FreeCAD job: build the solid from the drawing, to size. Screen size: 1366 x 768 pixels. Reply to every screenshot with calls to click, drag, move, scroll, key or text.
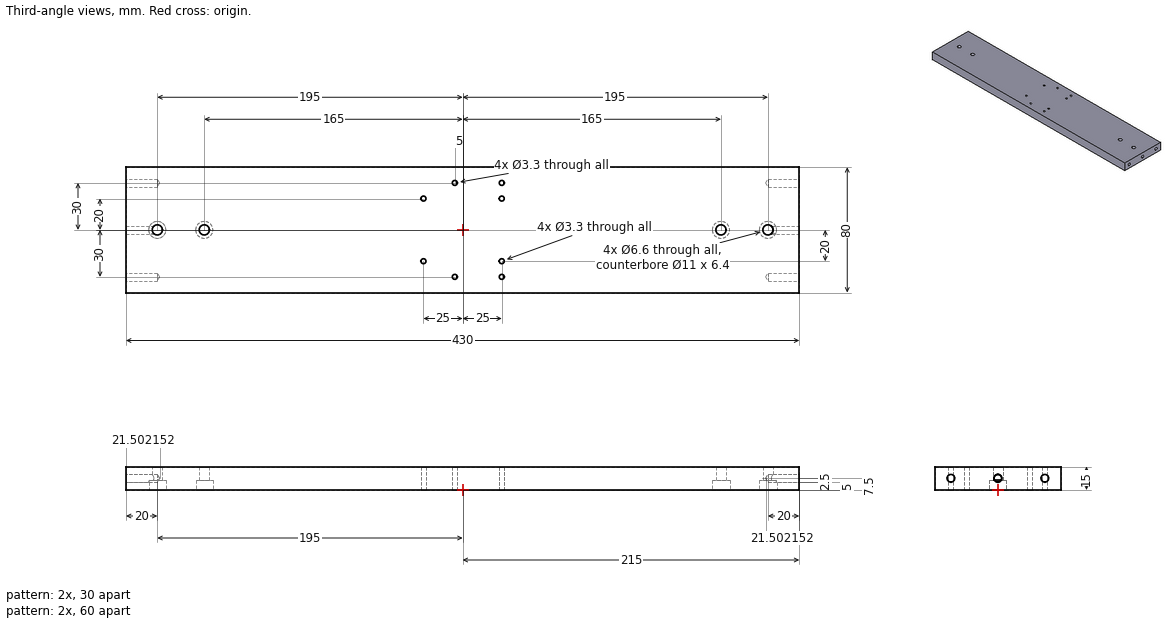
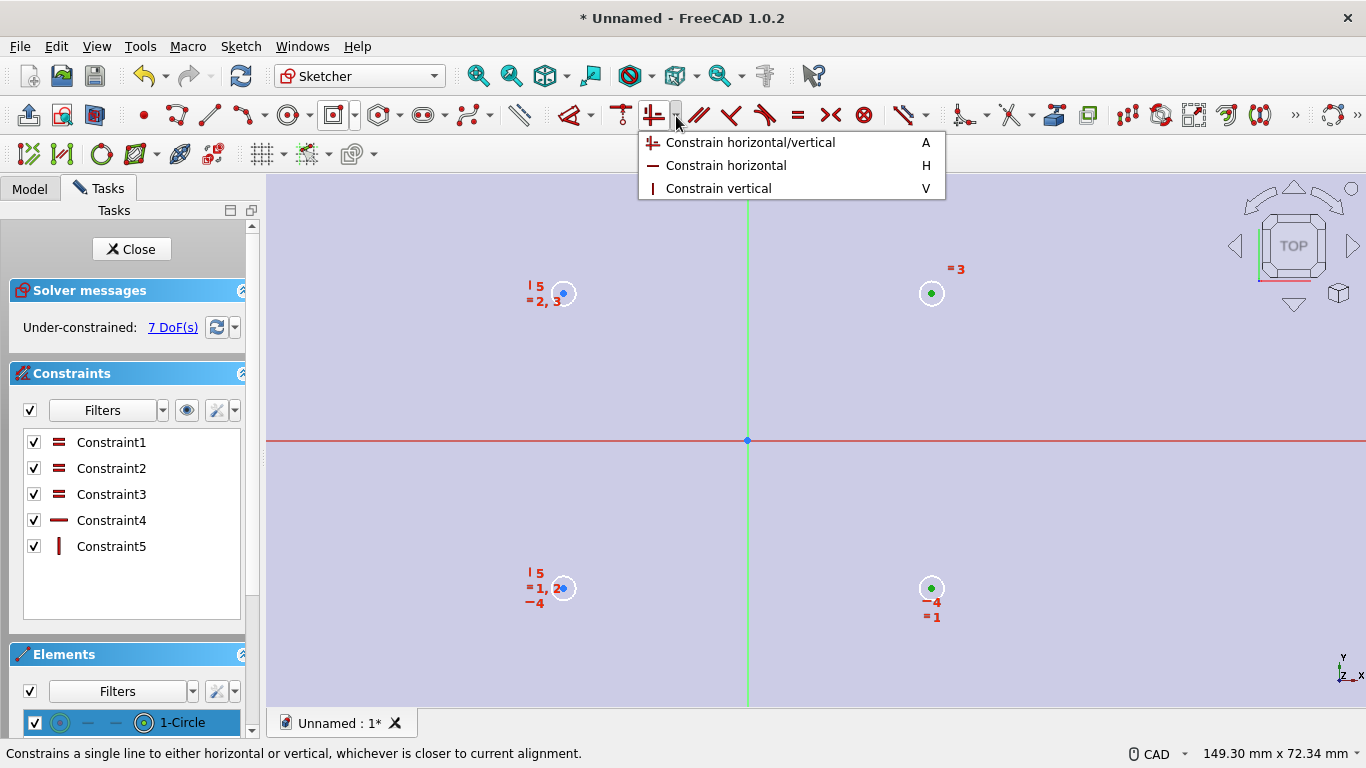
click(792, 188)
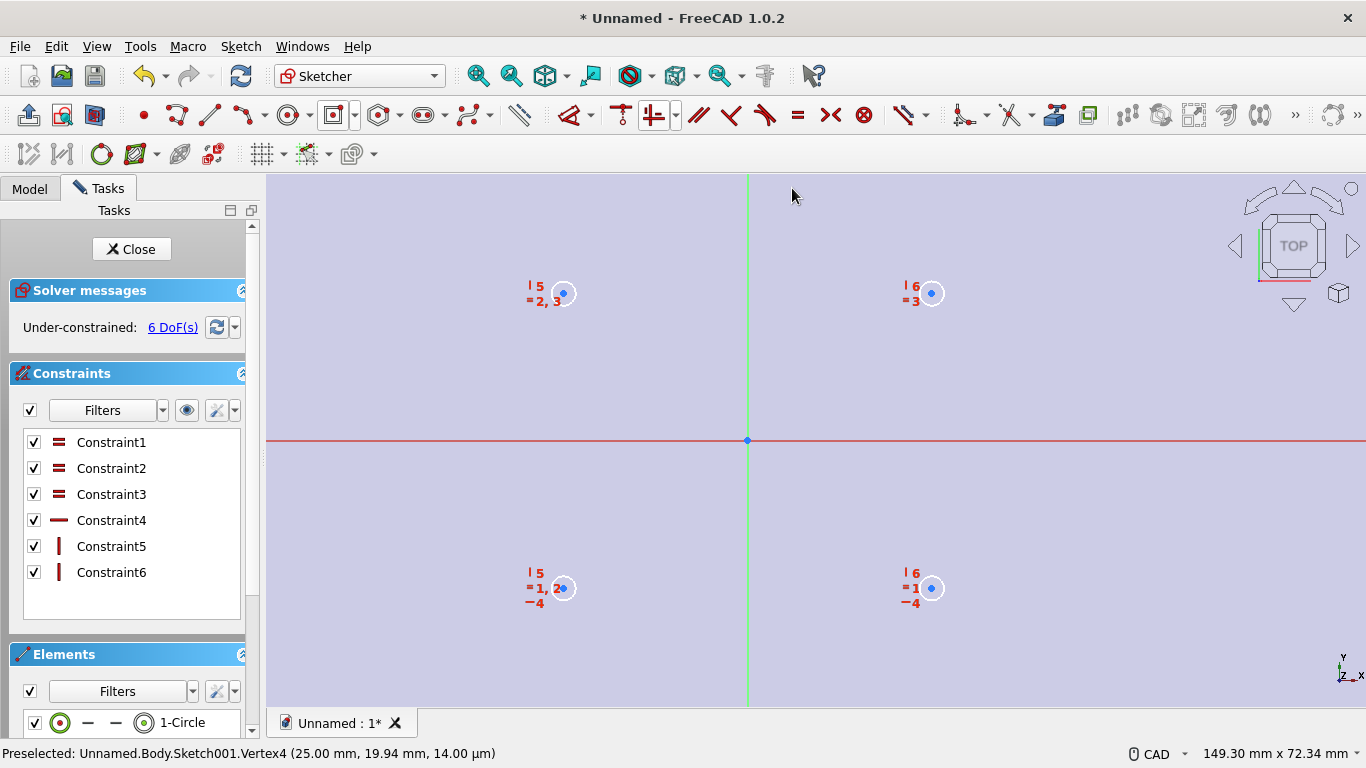
click(564, 294)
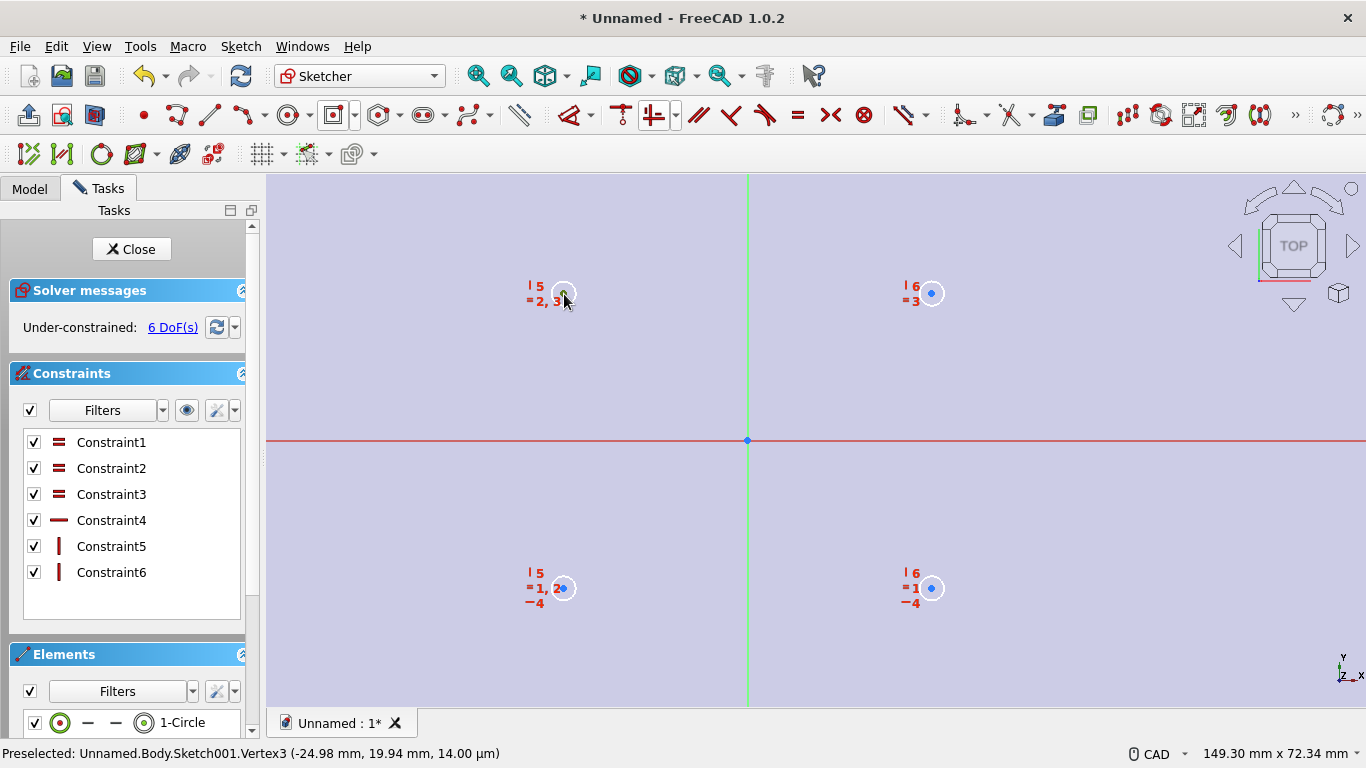
click(932, 294)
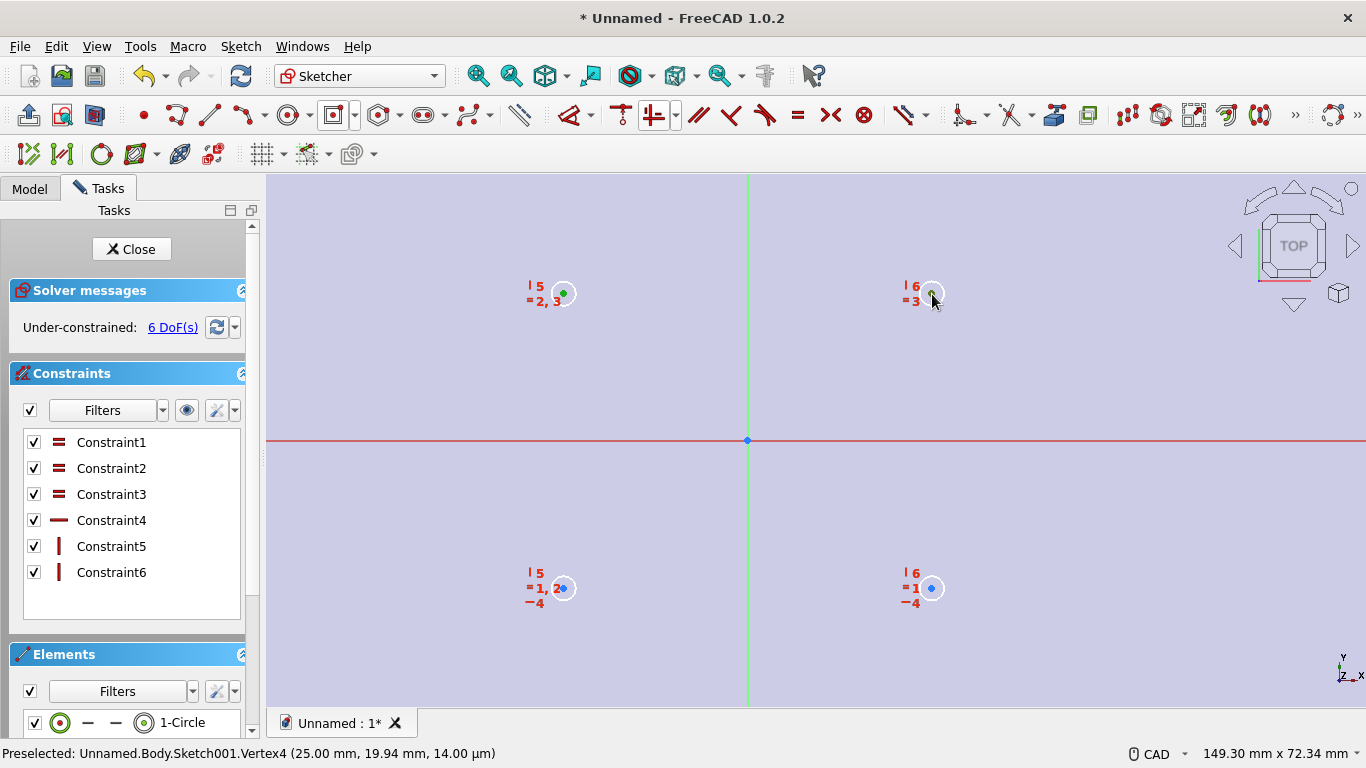
click(676, 116)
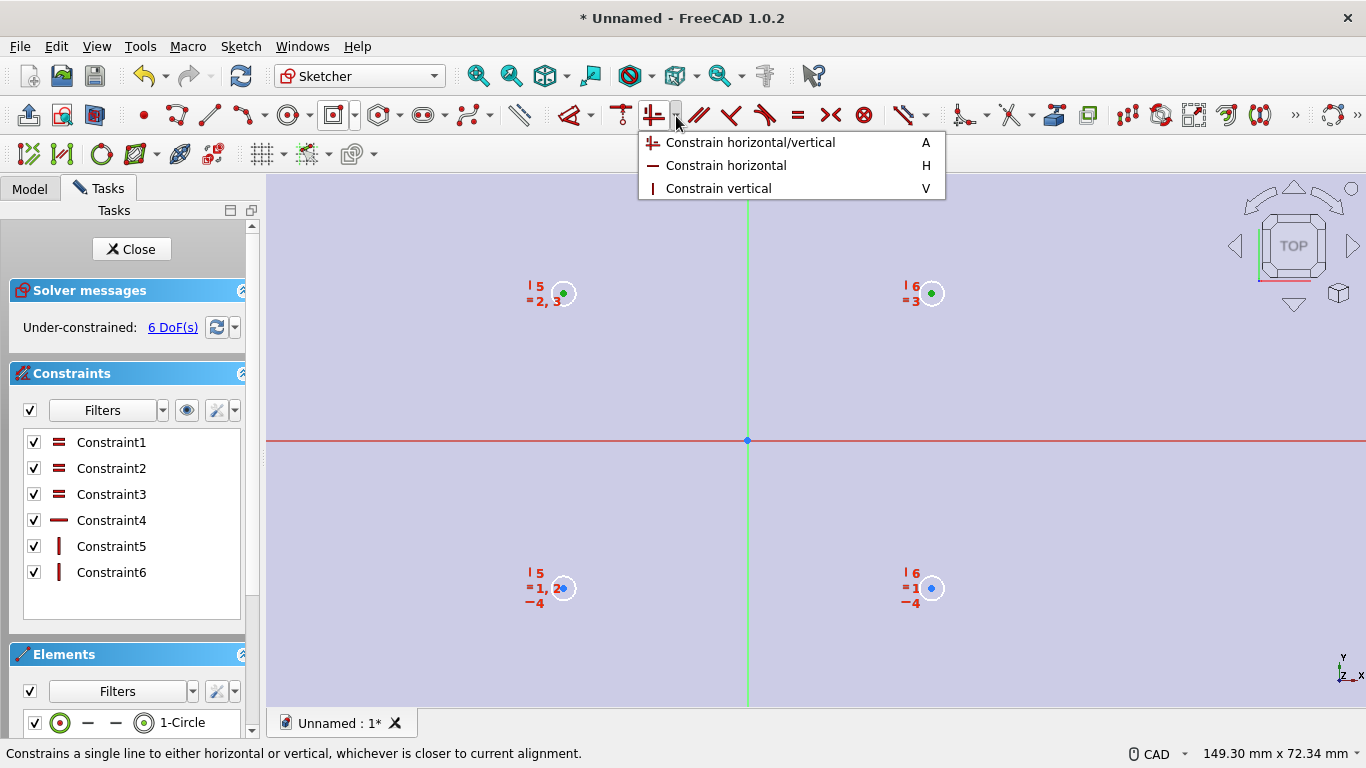
click(792, 166)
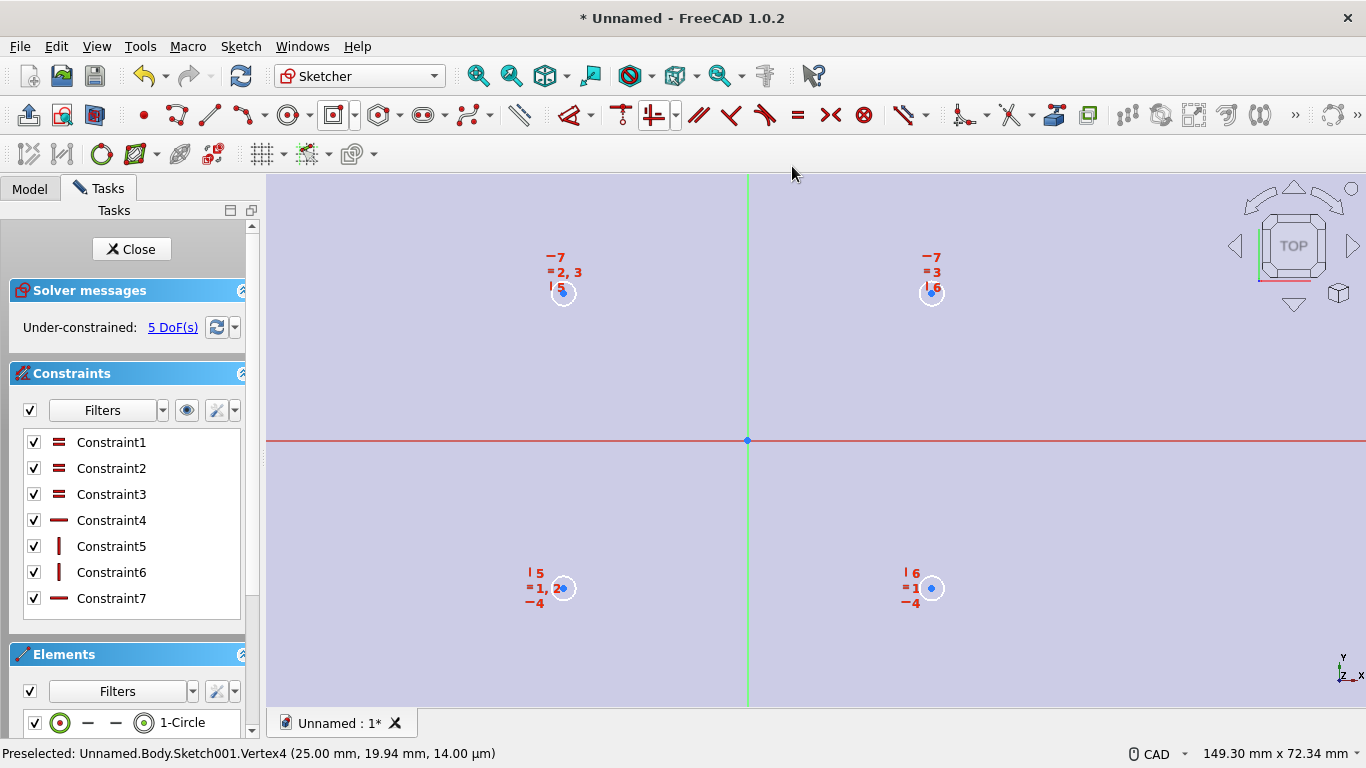
key(d)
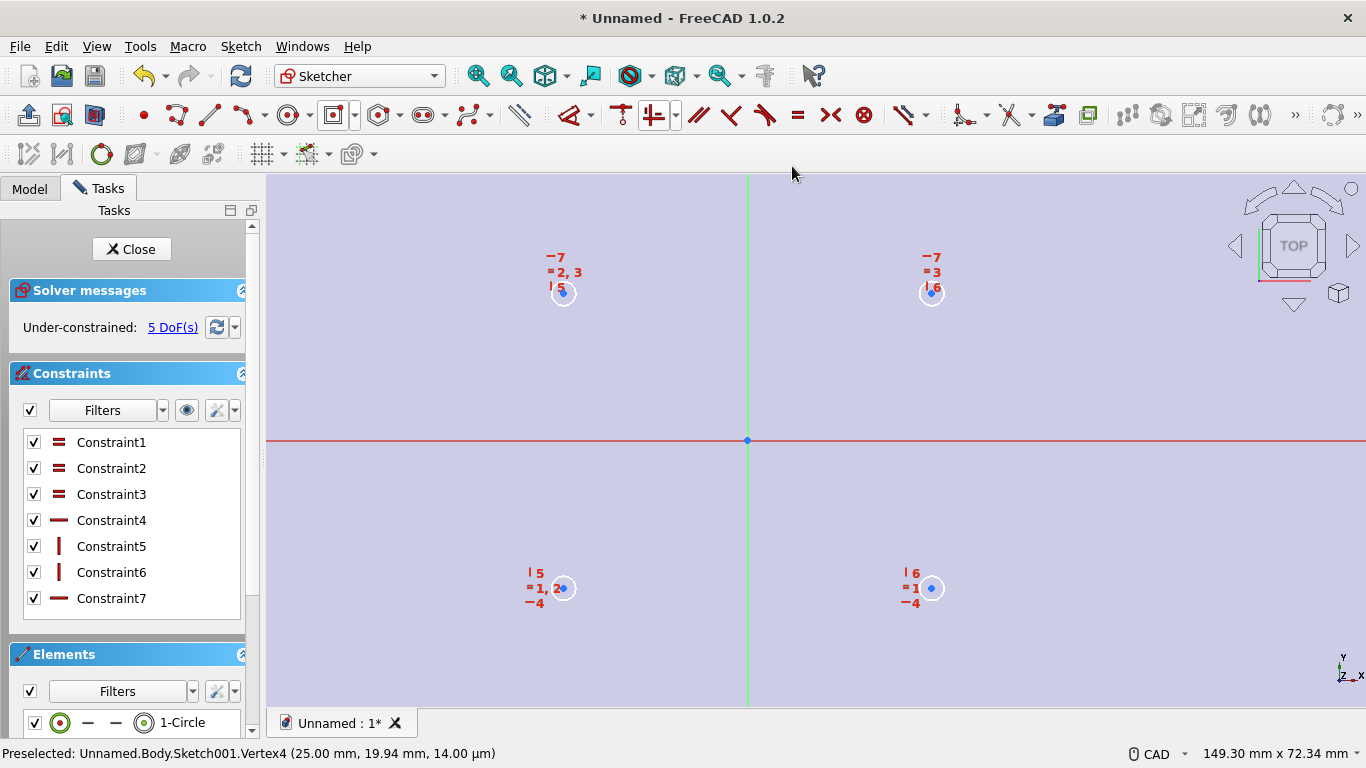
scroll(940, 580, up, 3)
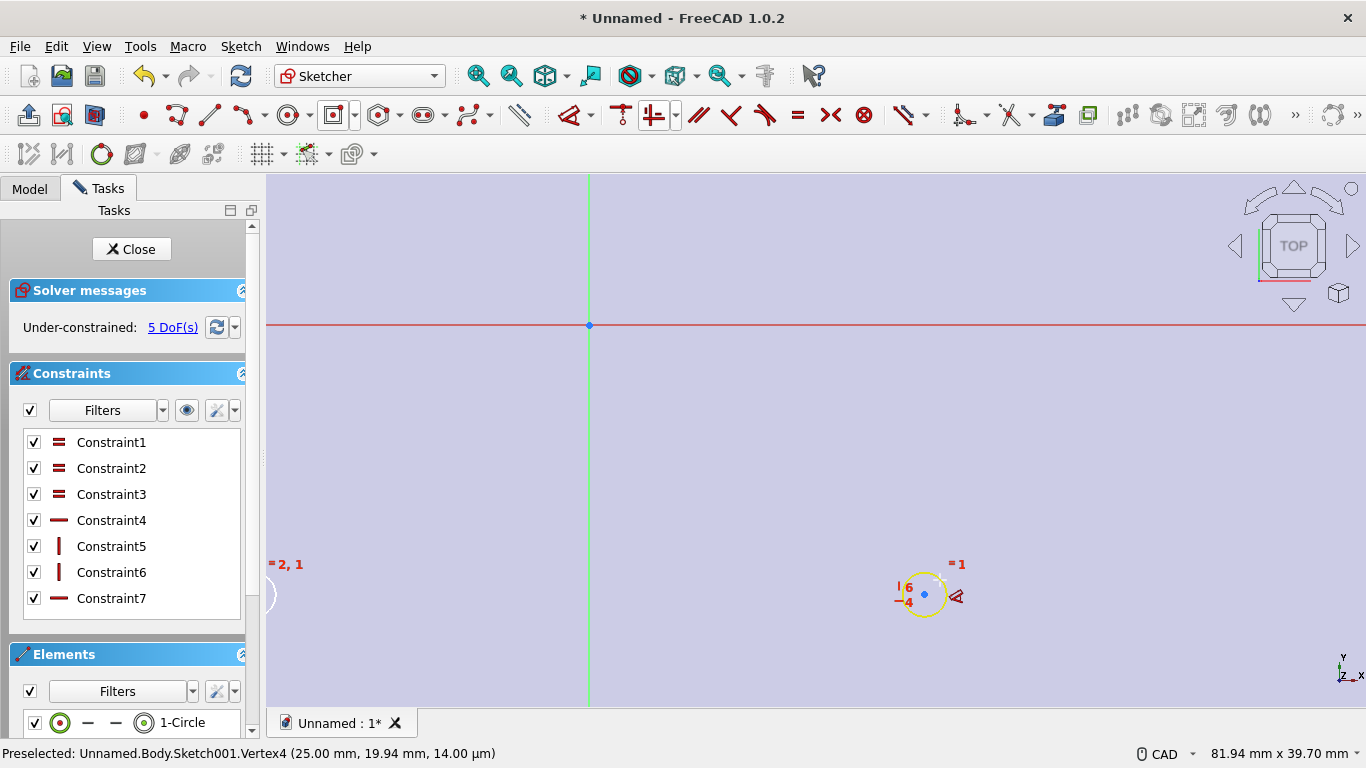
click(940, 579)
click(962, 556)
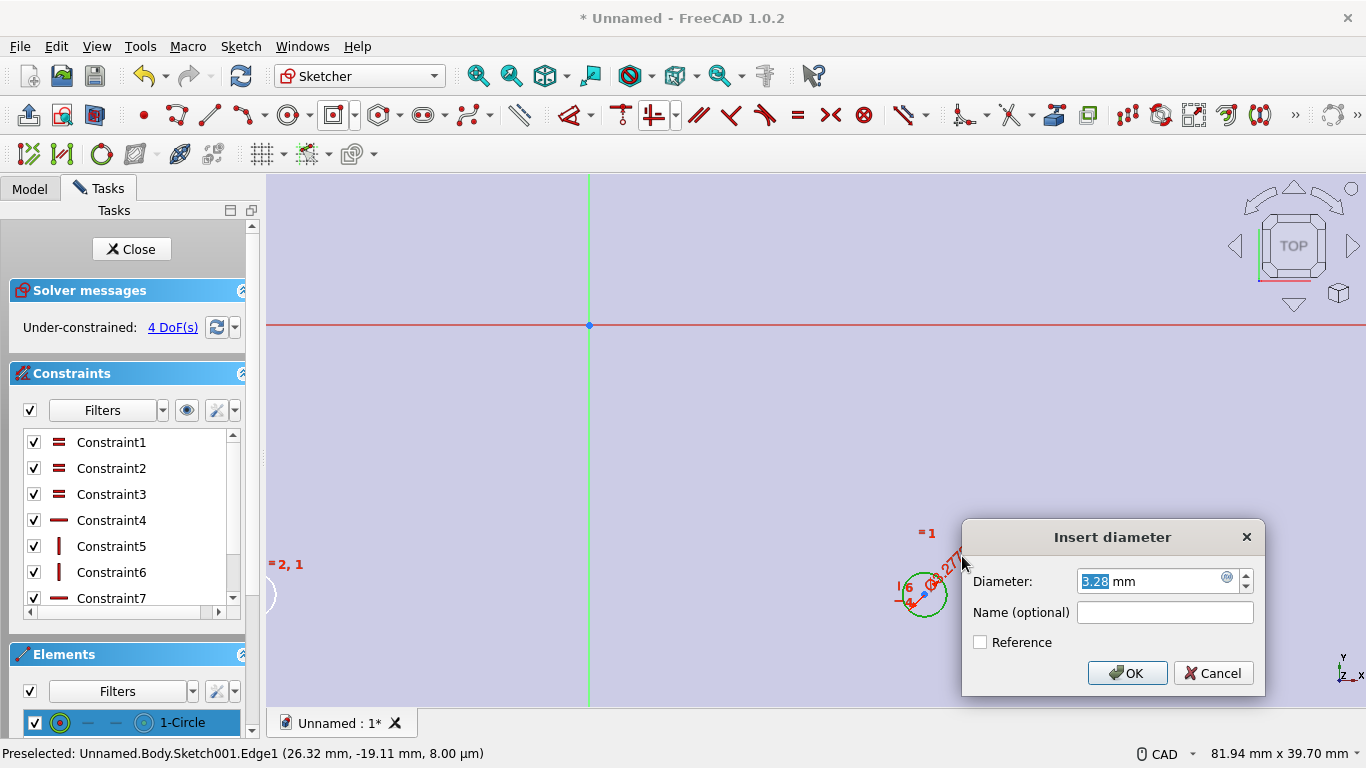
text(3.3)
key(Return)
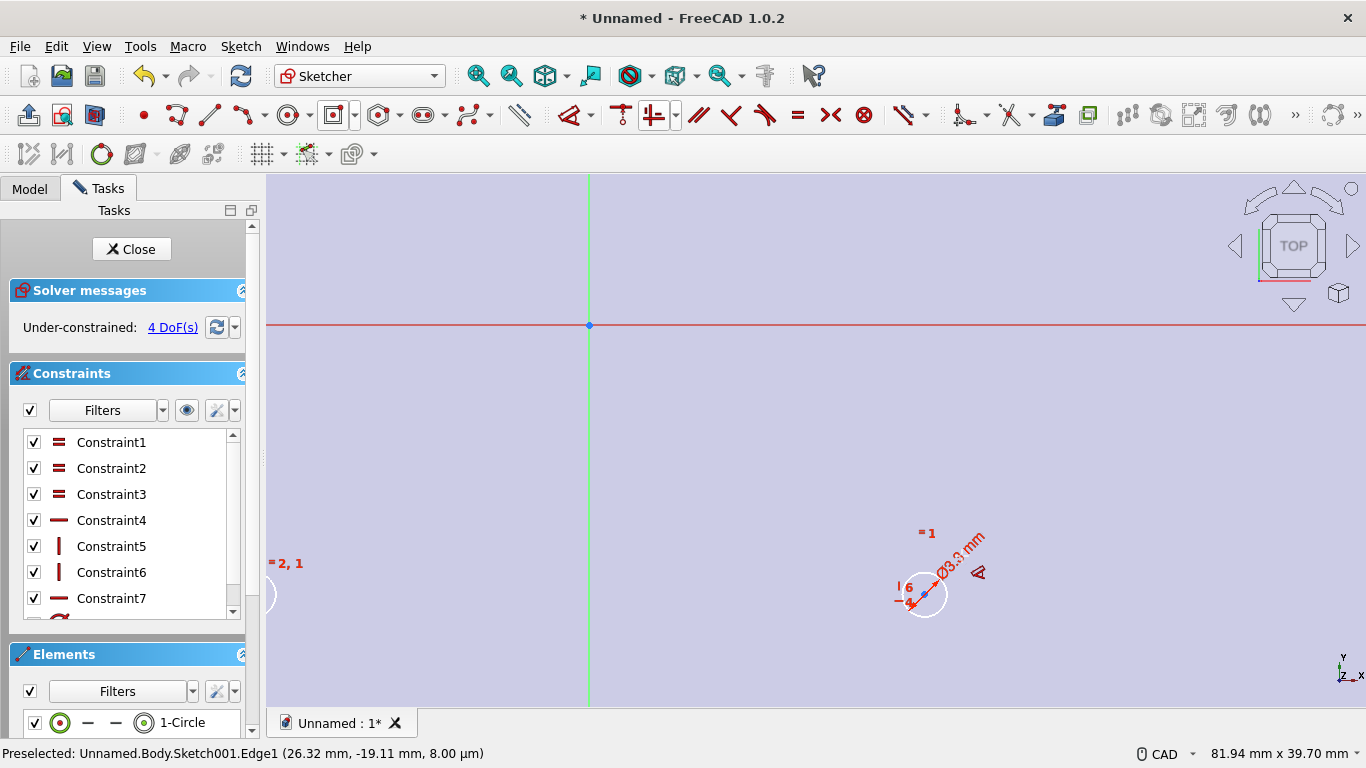
click(925, 595)
click(757, 629)